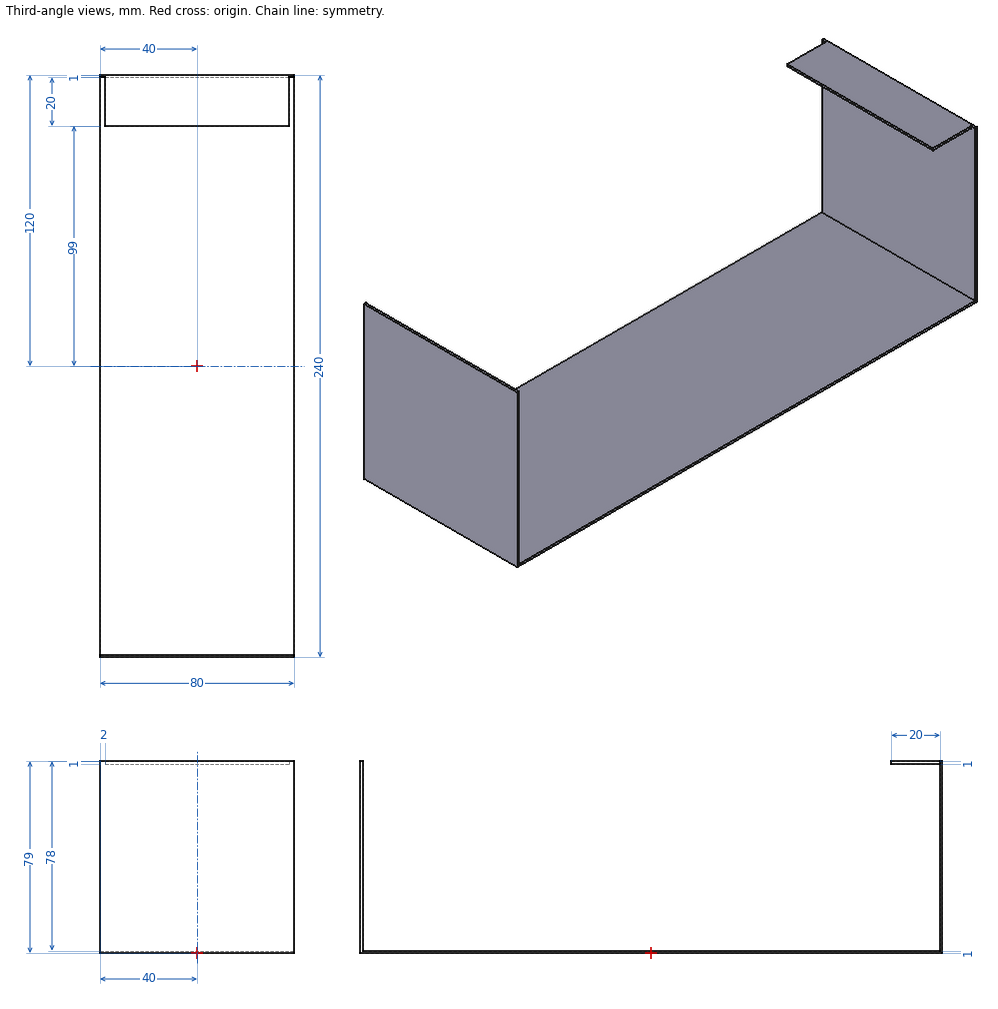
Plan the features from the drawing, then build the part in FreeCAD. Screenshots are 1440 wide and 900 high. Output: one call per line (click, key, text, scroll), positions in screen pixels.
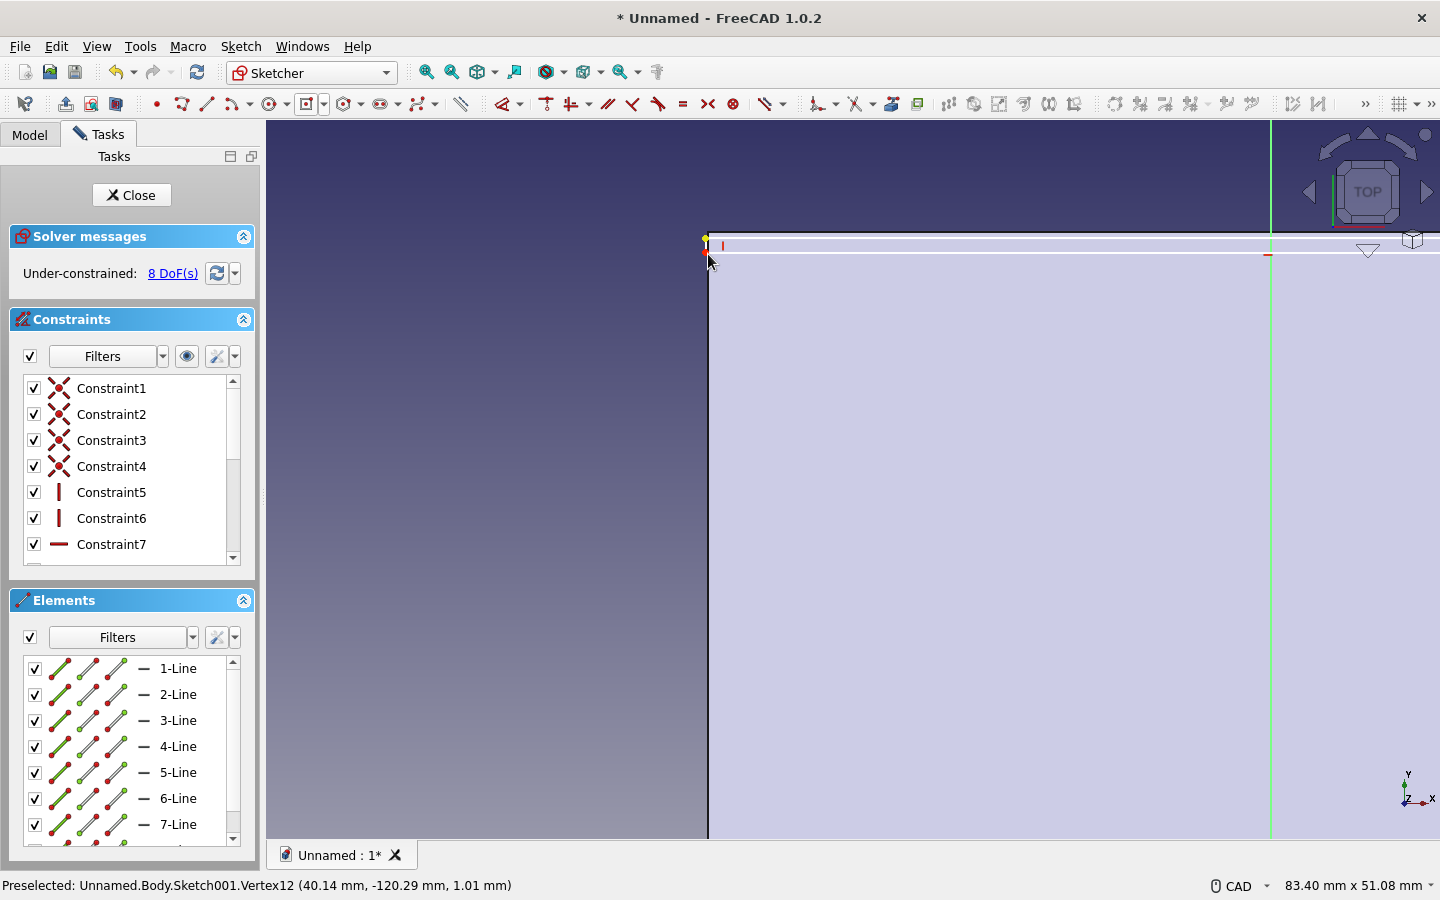
click(706, 253)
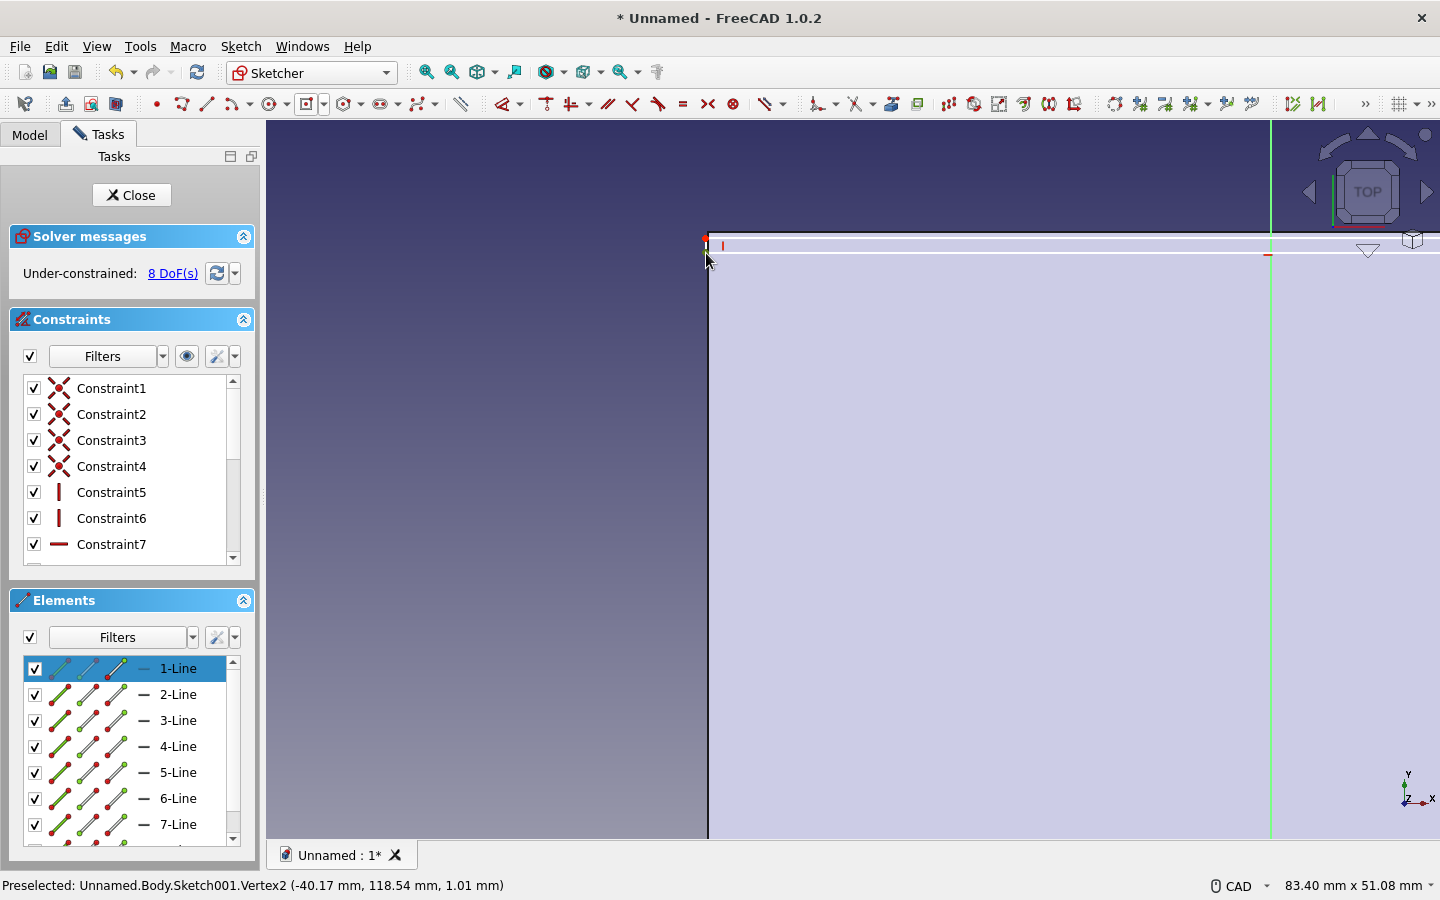
scroll(708, 254, down, 10)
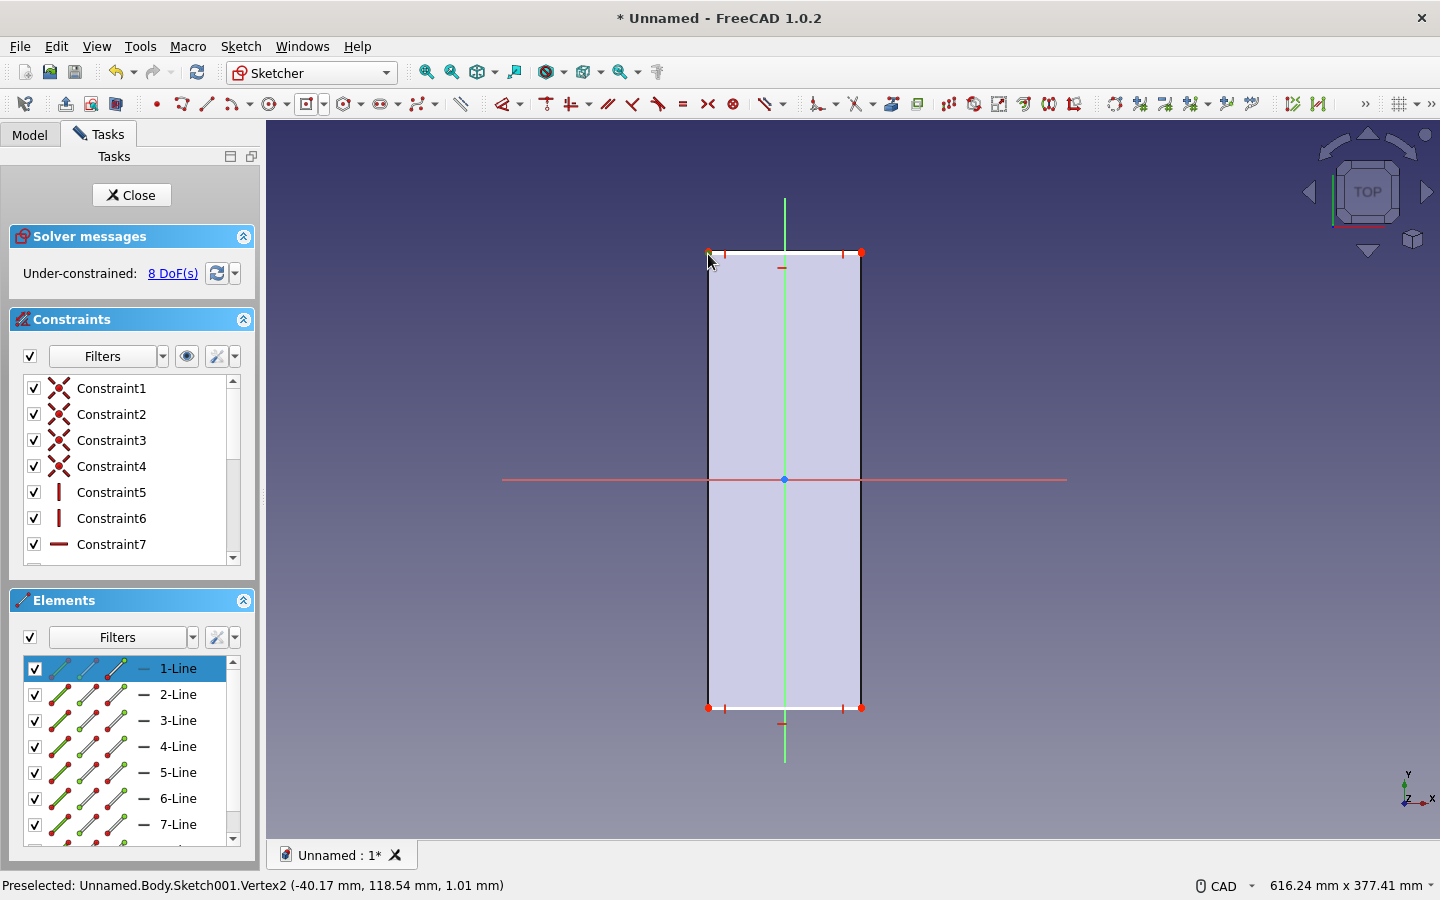
scroll(708, 708, up, 13)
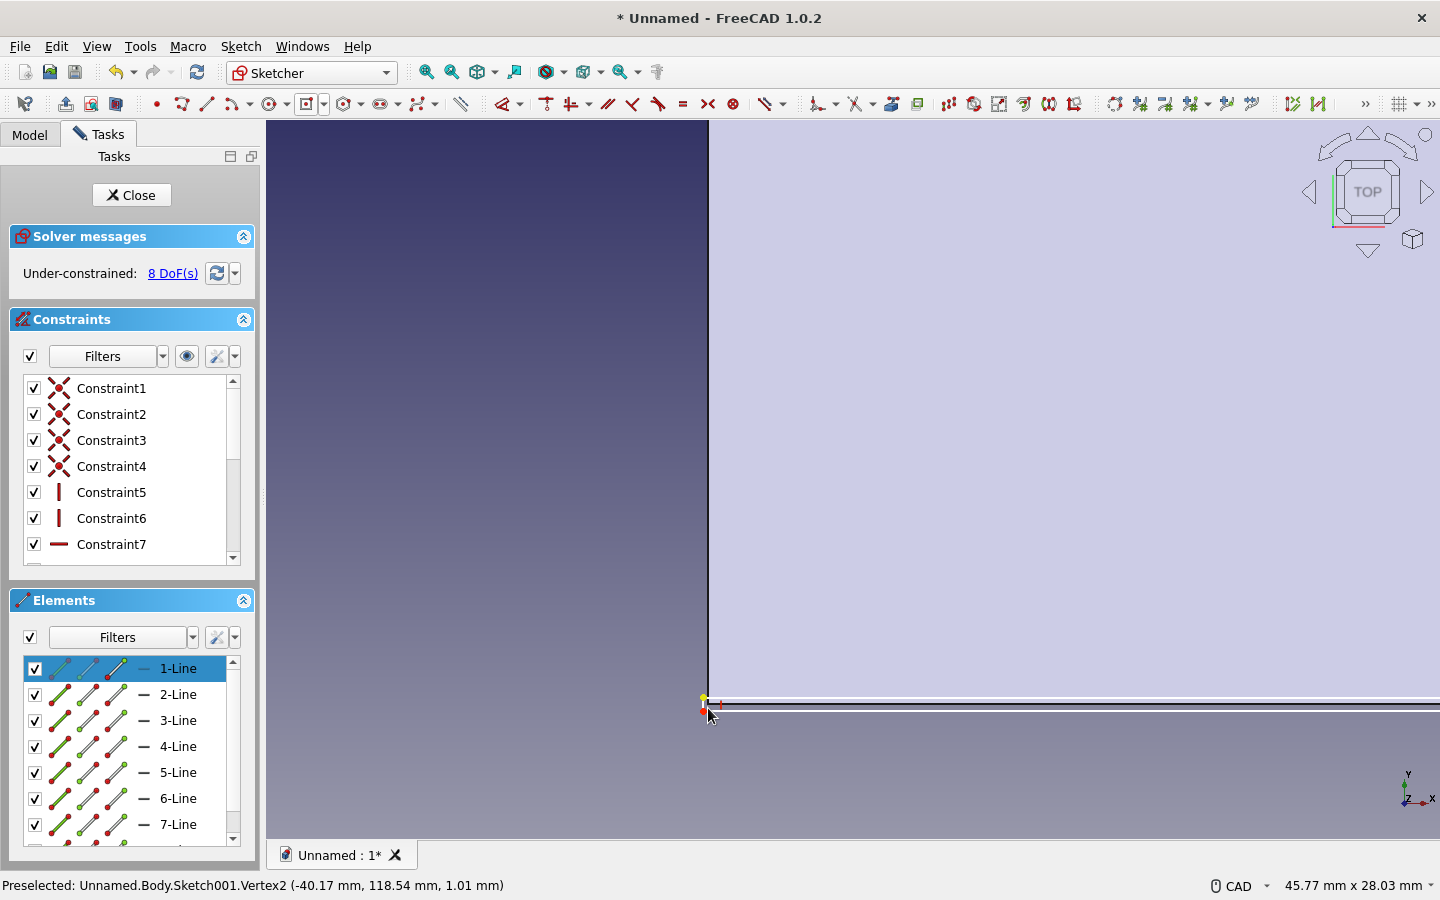
click(703, 698)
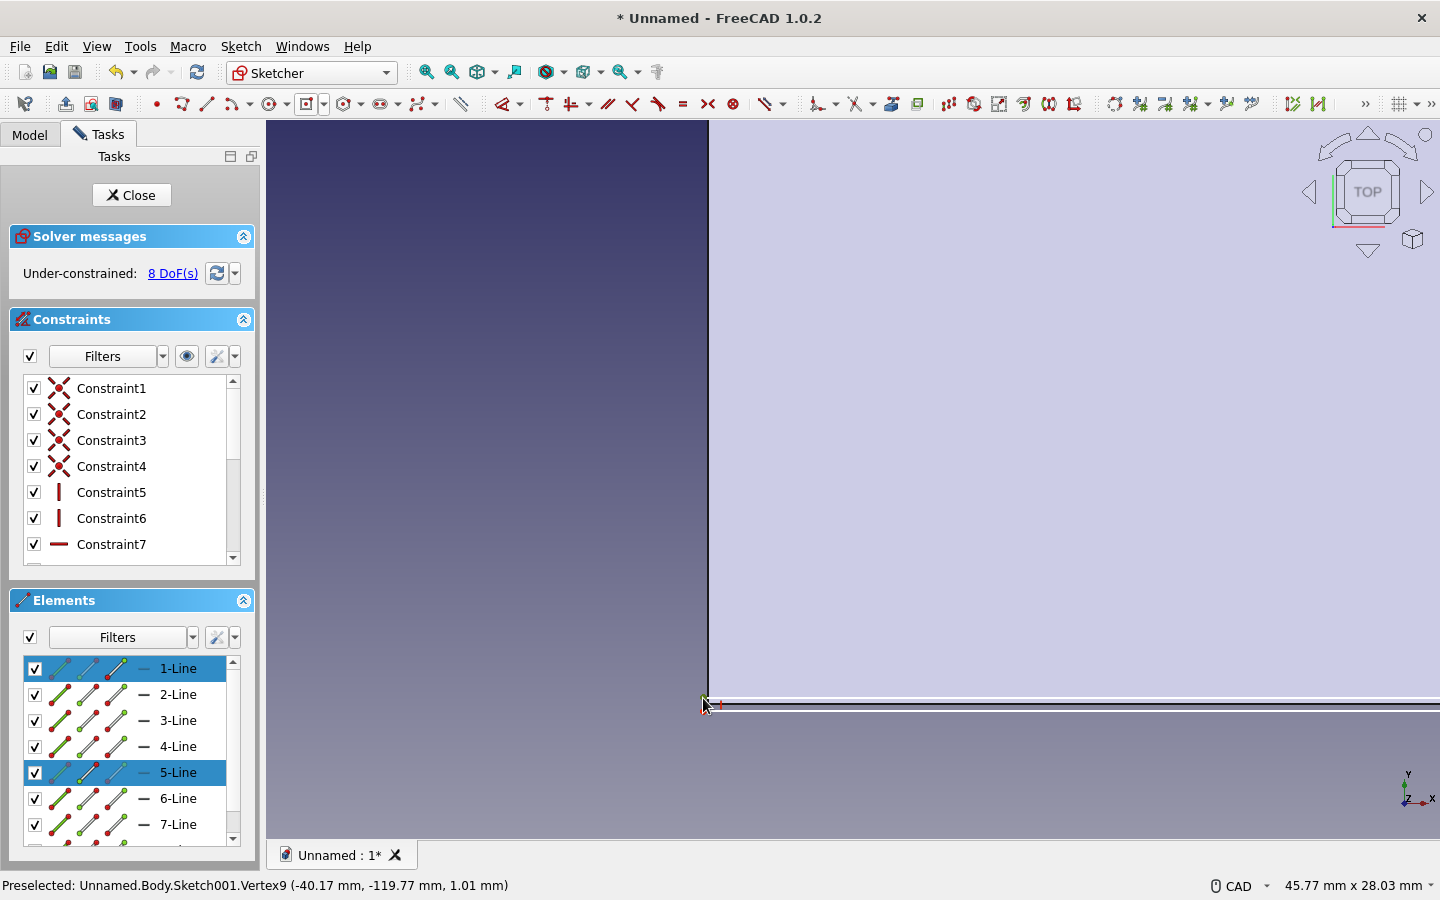
scroll(708, 708, down, 13)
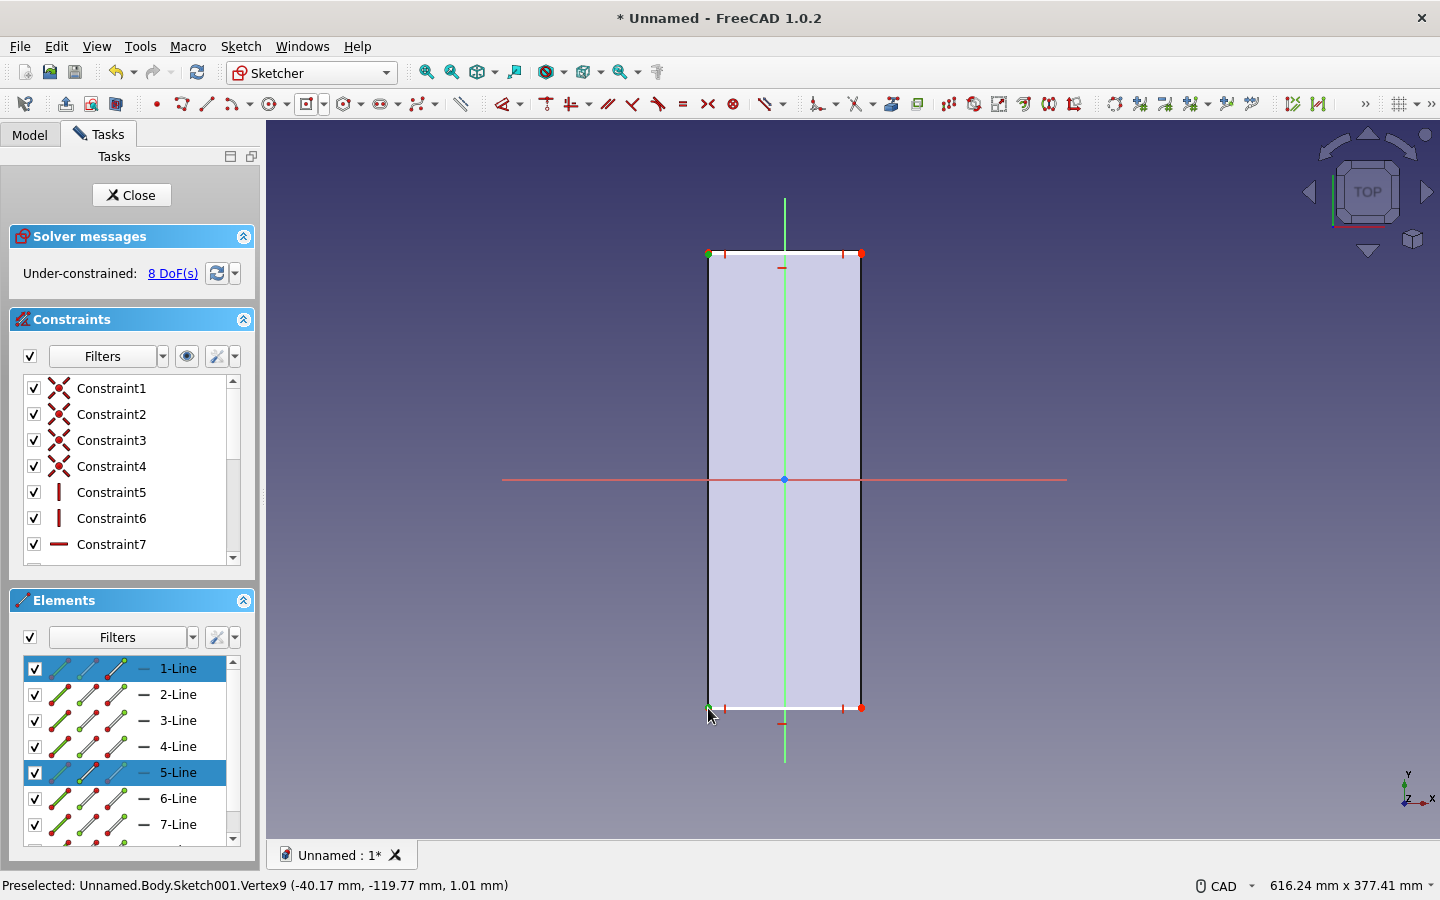
click(504, 480)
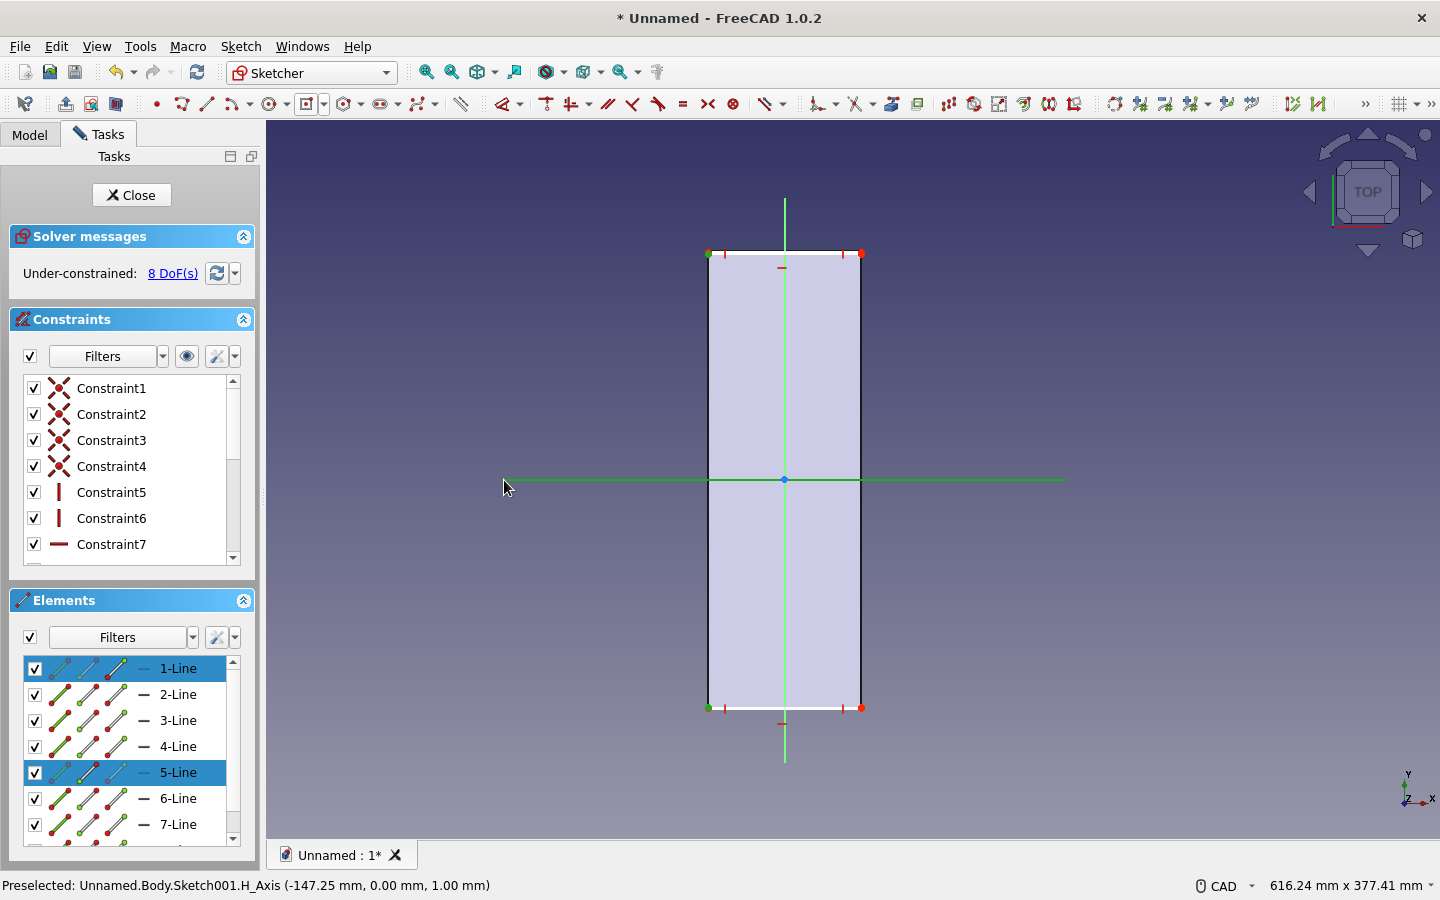
click(708, 104)